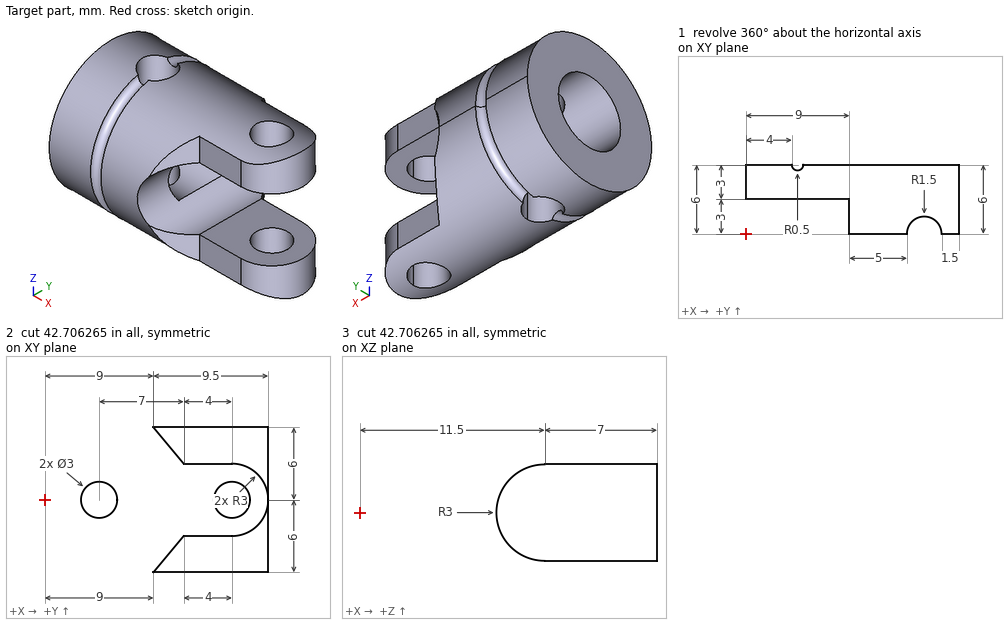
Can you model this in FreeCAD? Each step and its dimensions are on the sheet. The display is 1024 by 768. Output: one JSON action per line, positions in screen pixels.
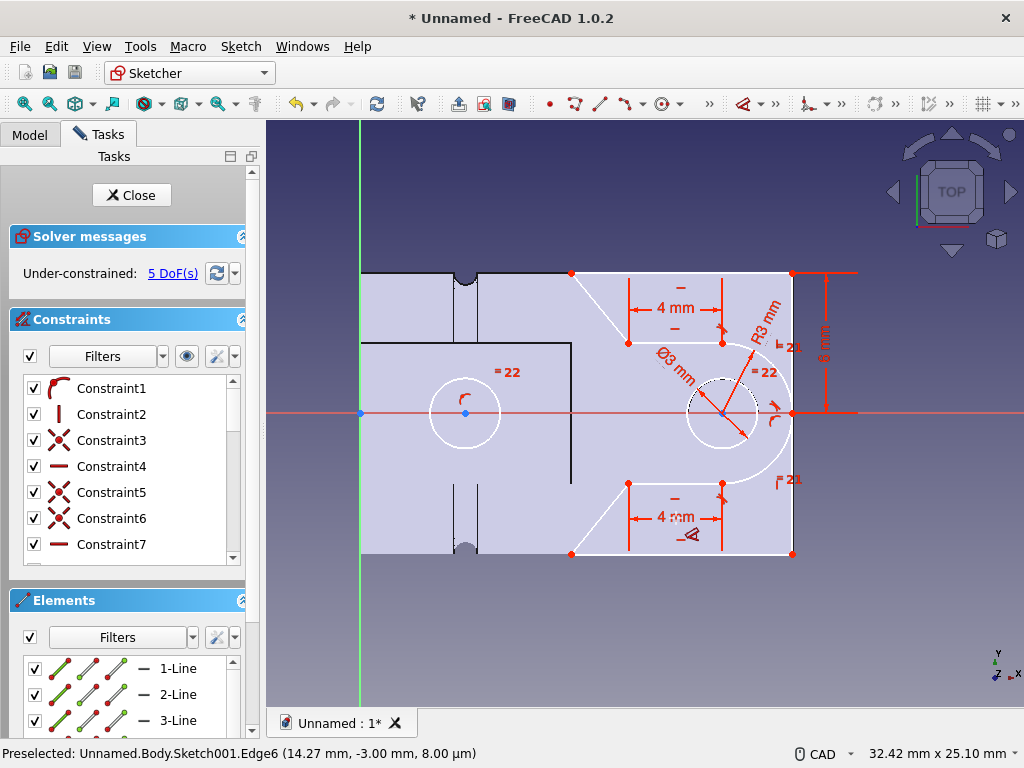
{"action": "left_click", "coordinate": [792, 512]}
{"action": "left_click", "coordinate": [826, 484]}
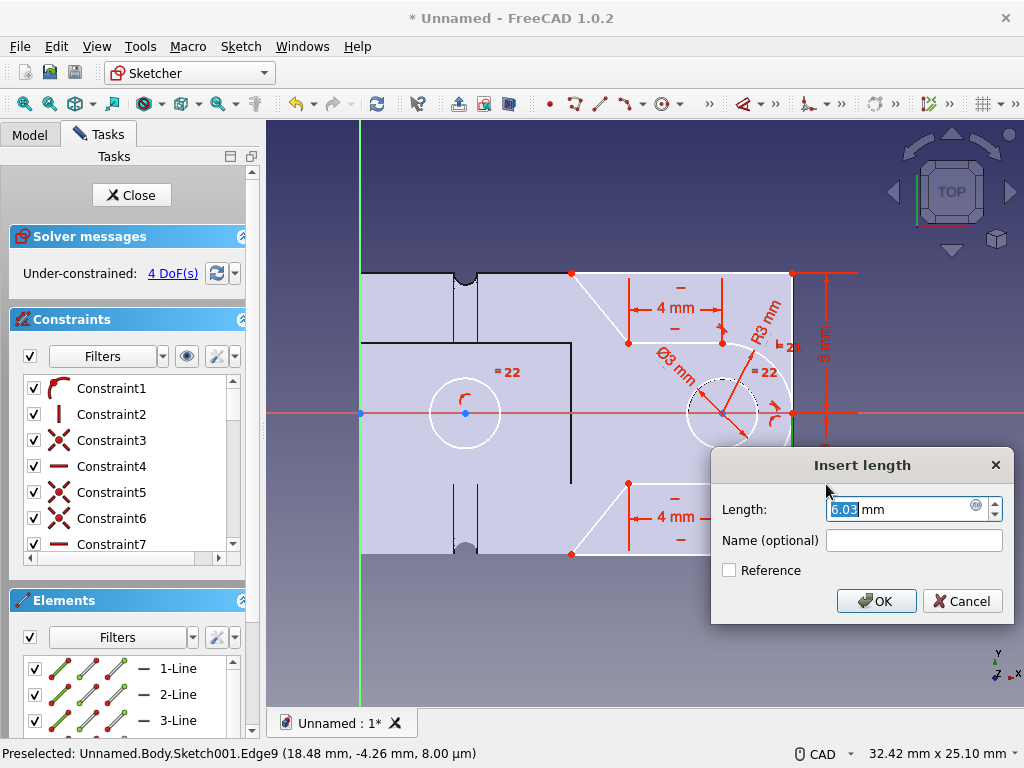
{"action": "type", "text": "6"}
{"action": "key", "text": "Return"}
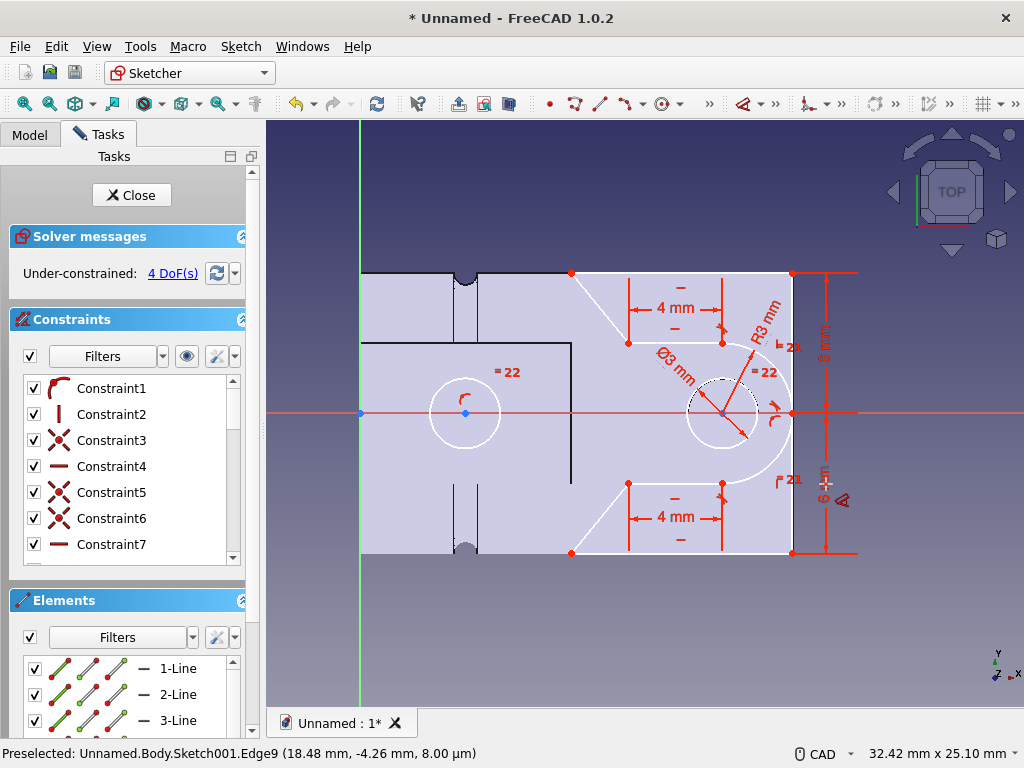
{"action": "left_click", "coordinate": [571, 273]}
{"action": "left_click", "coordinate": [466, 239]}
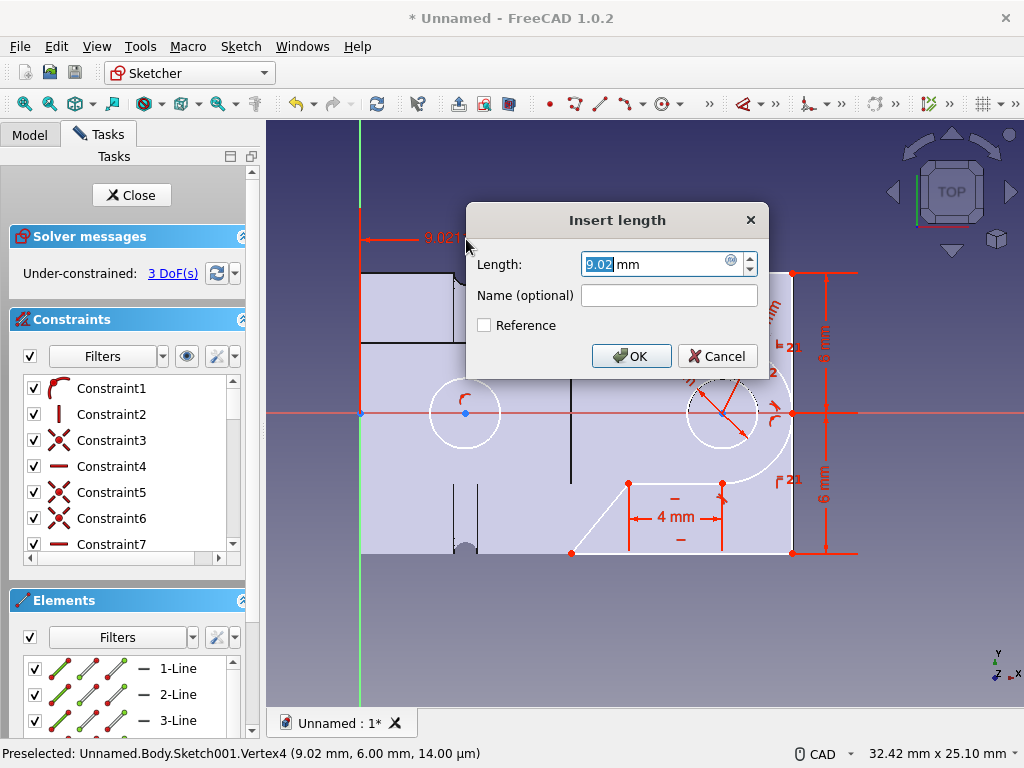
{"action": "type", "text": "9"}
{"action": "key", "text": "Return"}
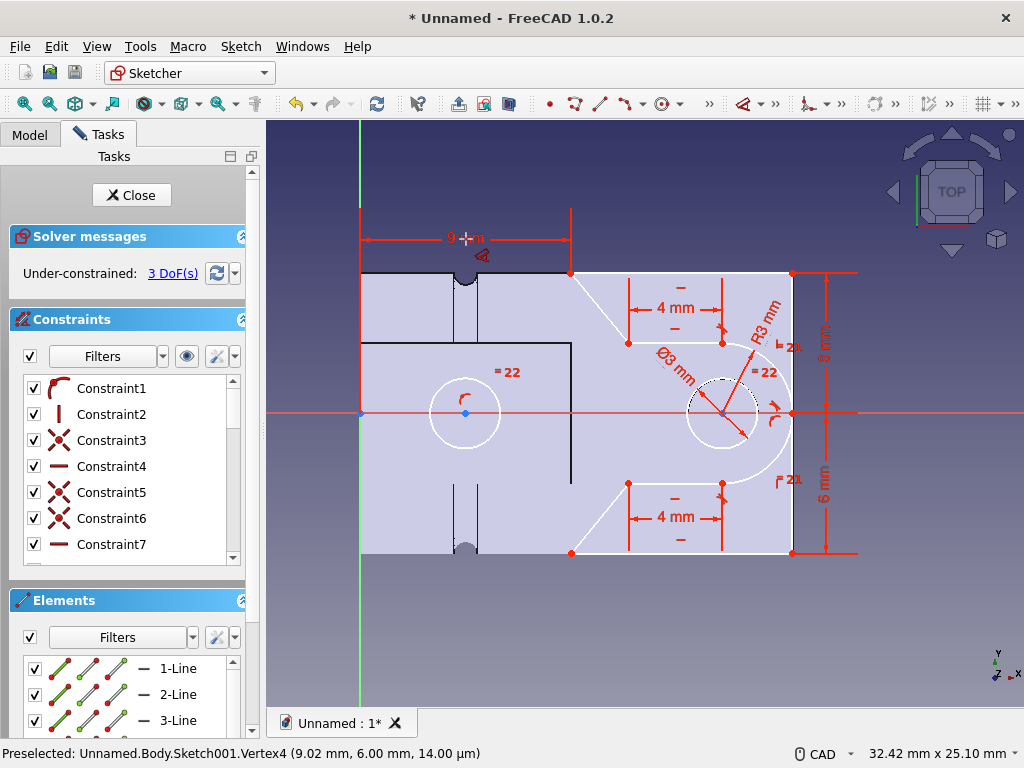
{"action": "left_click", "coordinate": [571, 554]}
{"action": "left_click", "coordinate": [466, 588]}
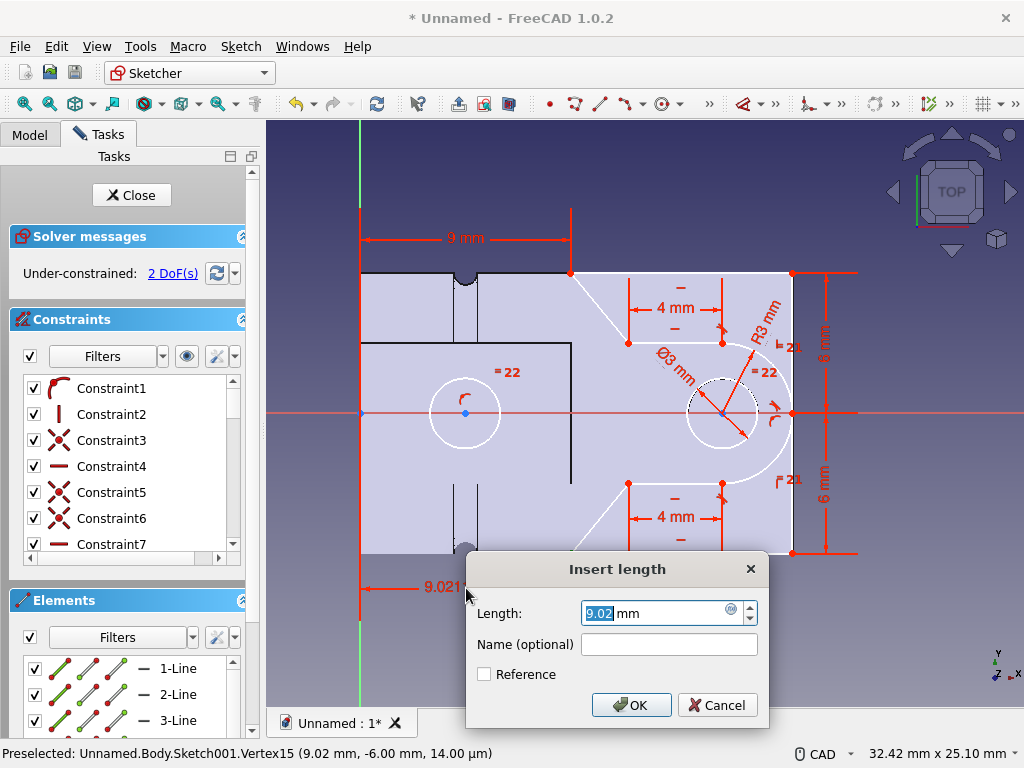
{"action": "type", "text": "9"}
{"action": "key", "text": "Return"}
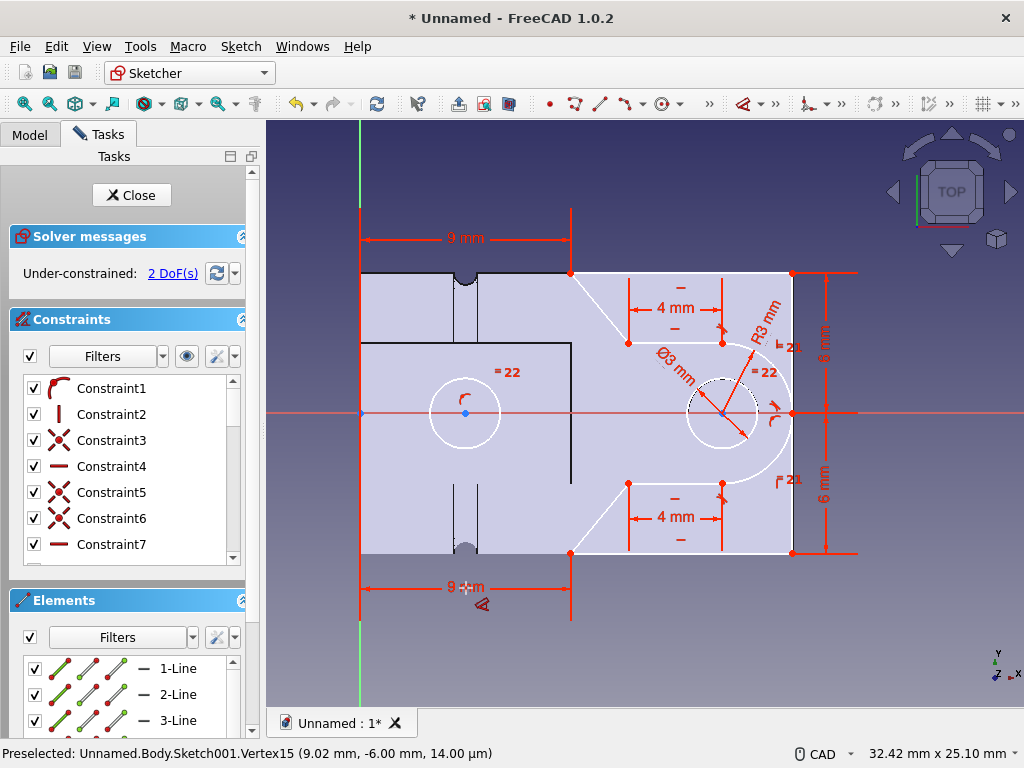
{"action": "left_click", "coordinate": [629, 343]}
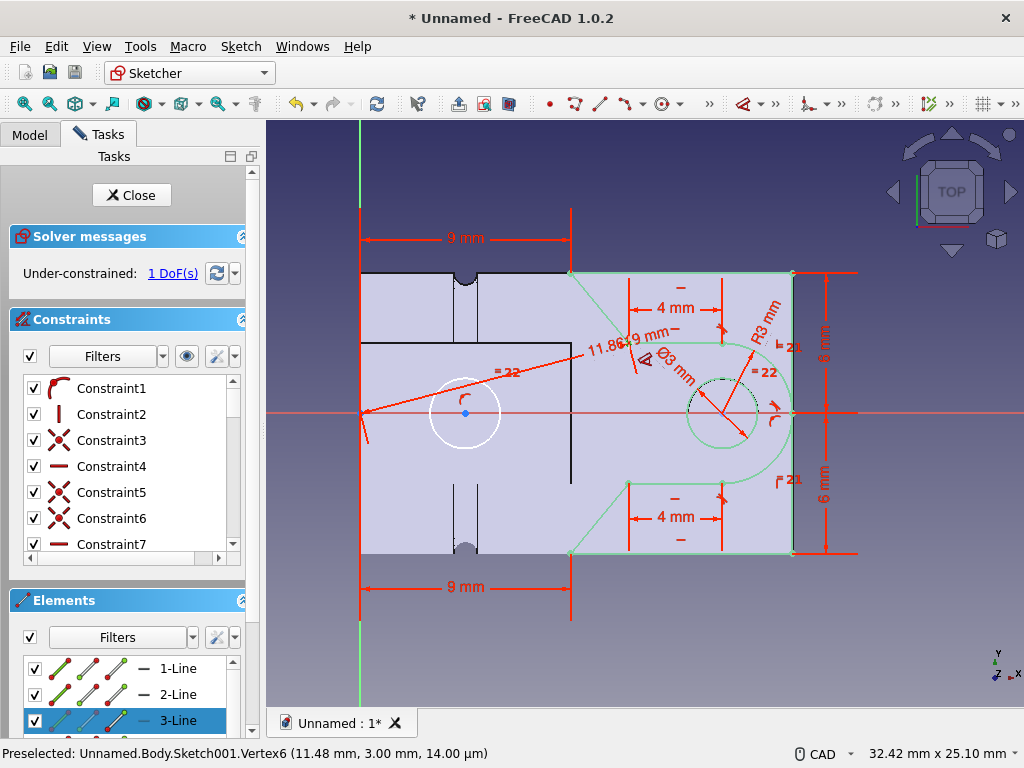
{"action": "left_click", "coordinate": [465, 413]}
{"action": "left_click", "coordinate": [547, 309]}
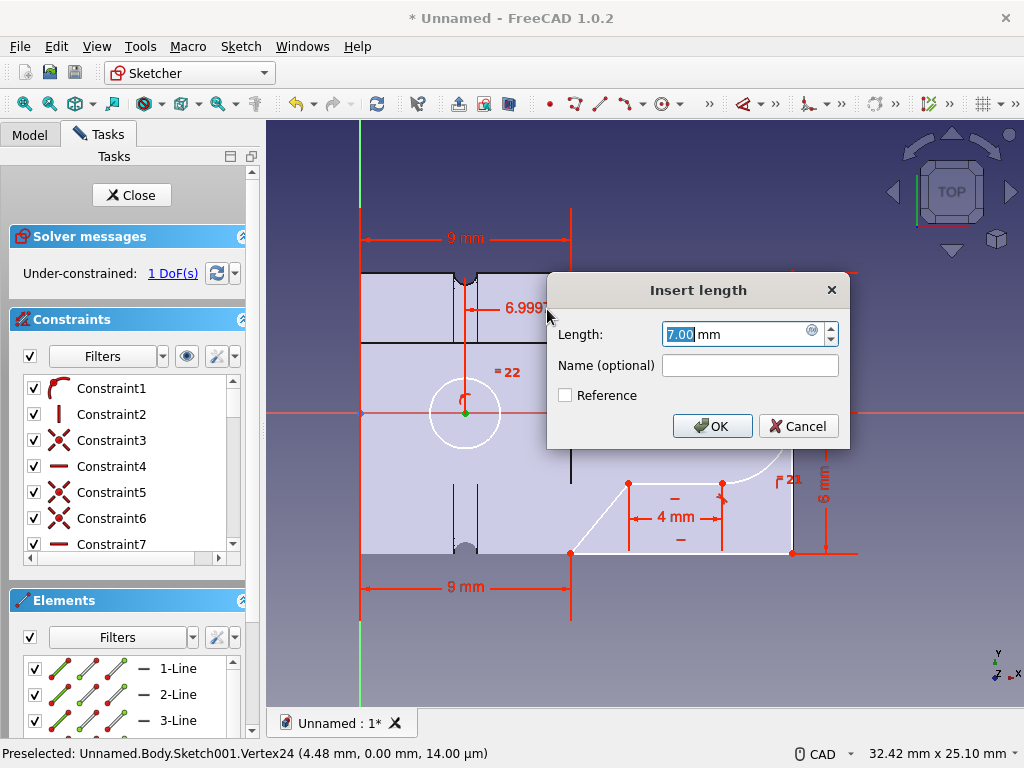
{"action": "type", "text": "7"}
{"action": "key", "text": "Return"}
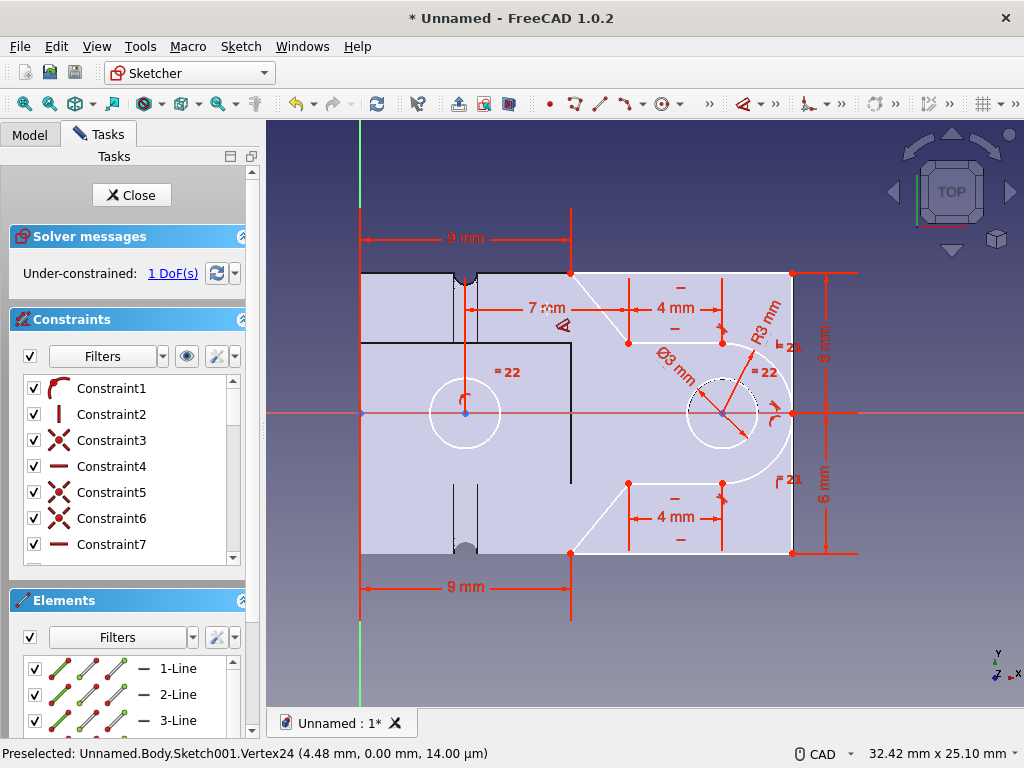
{"action": "left_click", "coordinate": [726, 273]}
{"action": "left_click", "coordinate": [682, 239]}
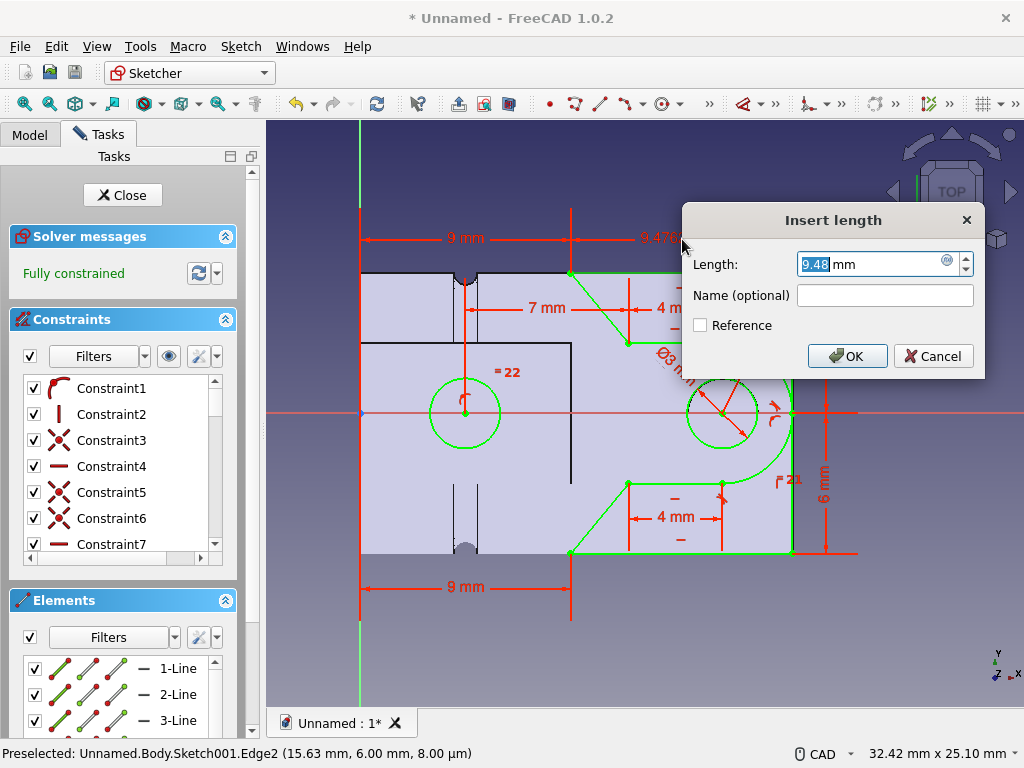
{"action": "type", "text": "9.5"}
{"action": "key", "text": "Return"}
{"action": "key", "text": "Escape"}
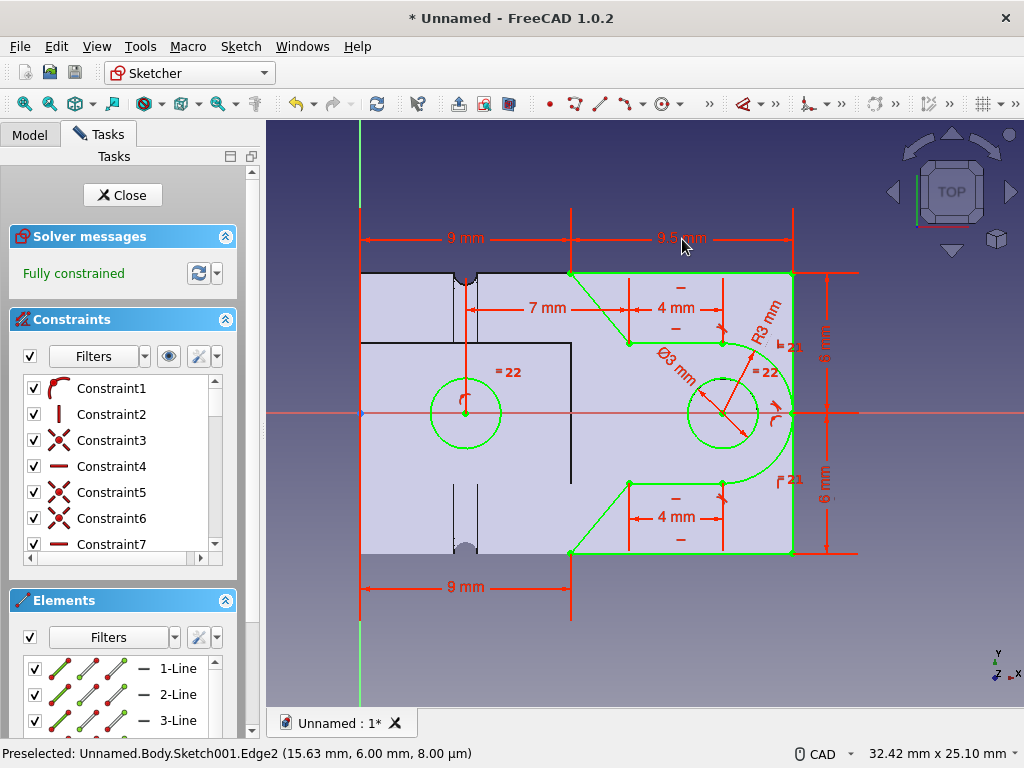
{"action": "left_click", "coordinate": [123, 195]}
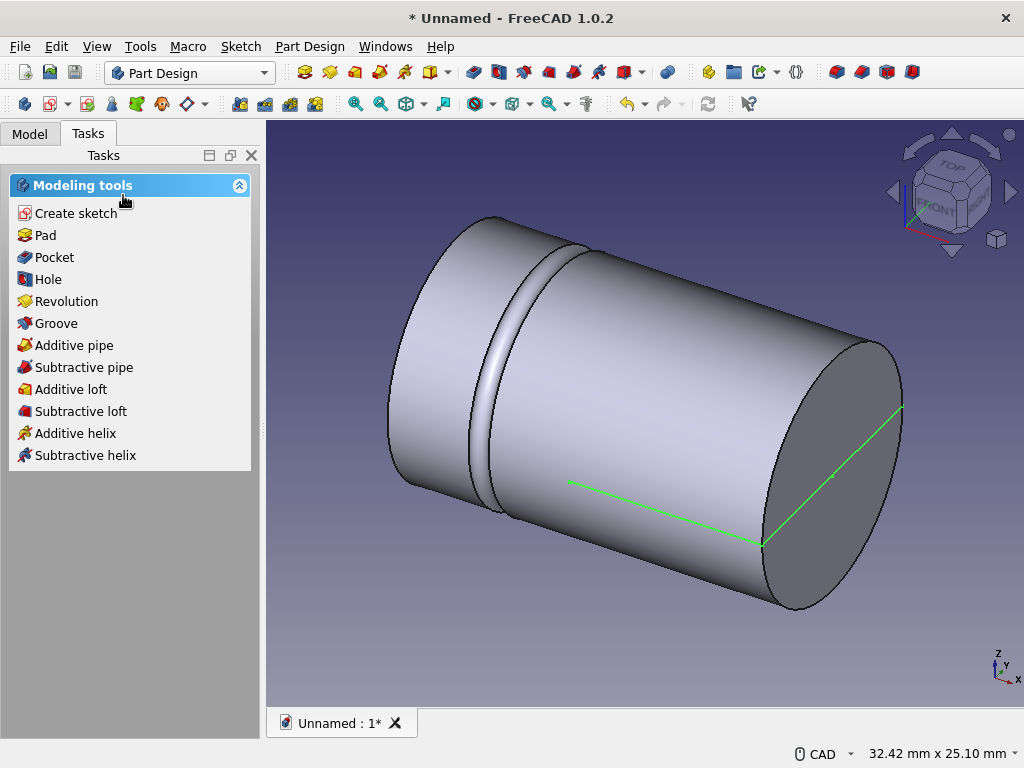
{"action": "left_click", "coordinate": [474, 72]}